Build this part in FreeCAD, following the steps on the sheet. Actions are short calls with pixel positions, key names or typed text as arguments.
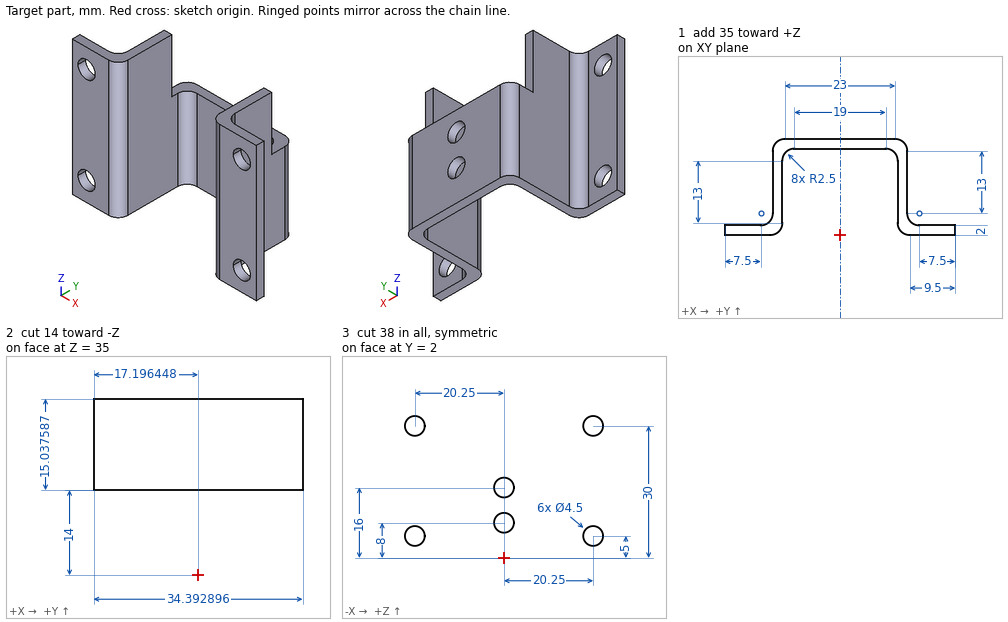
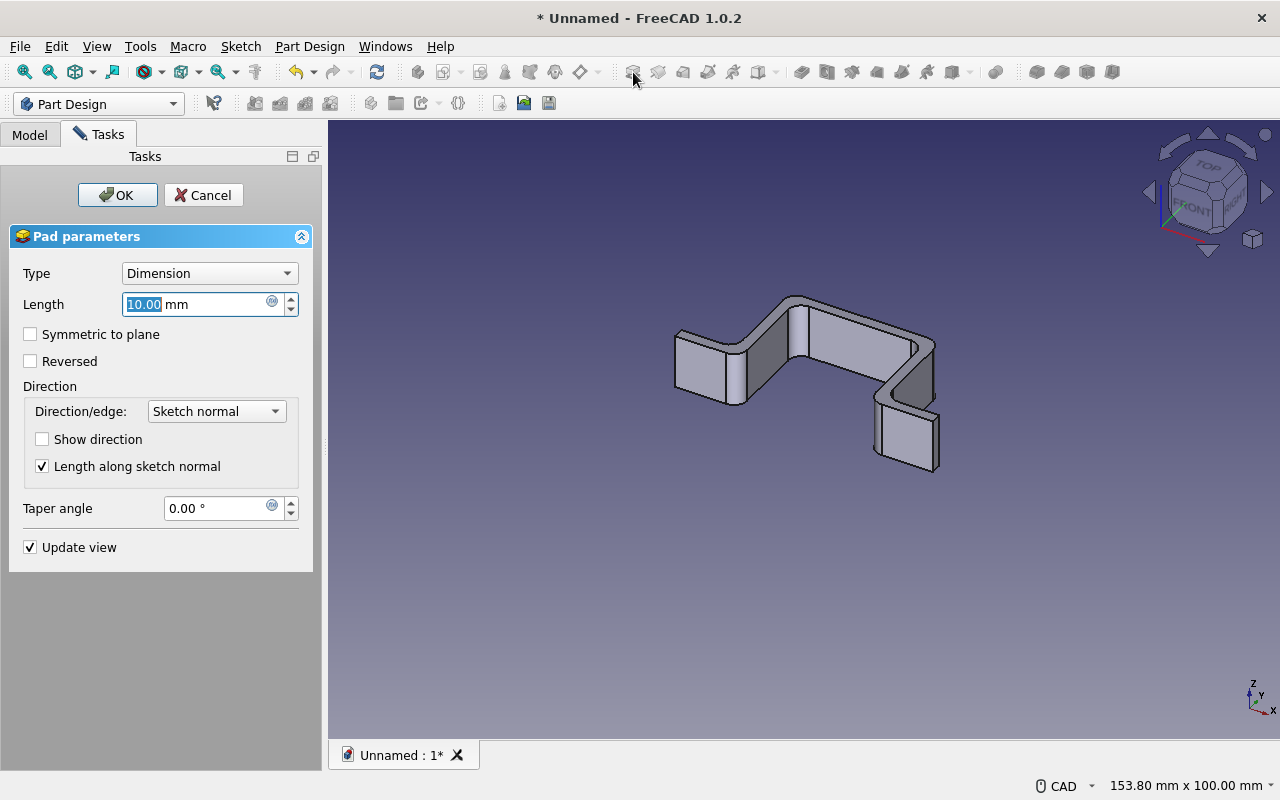
text(35)
key(Tab)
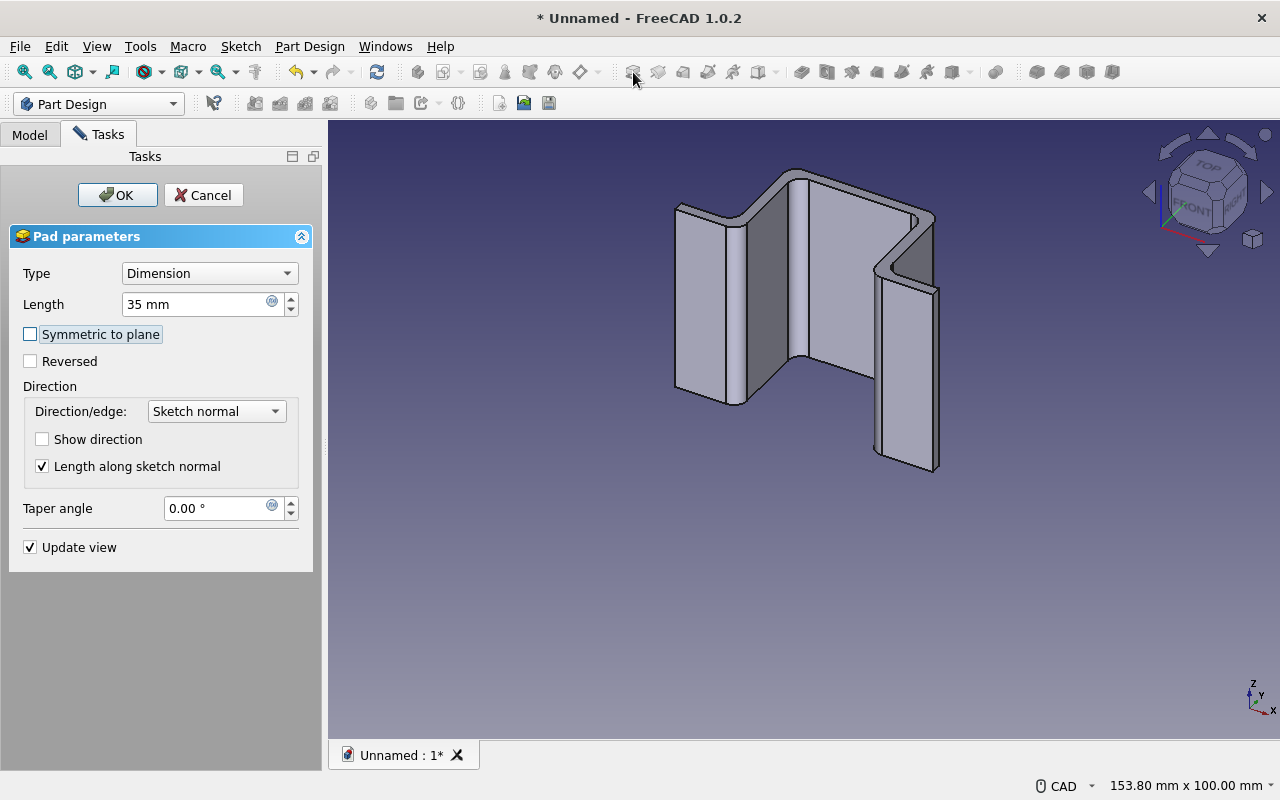
click(118, 195)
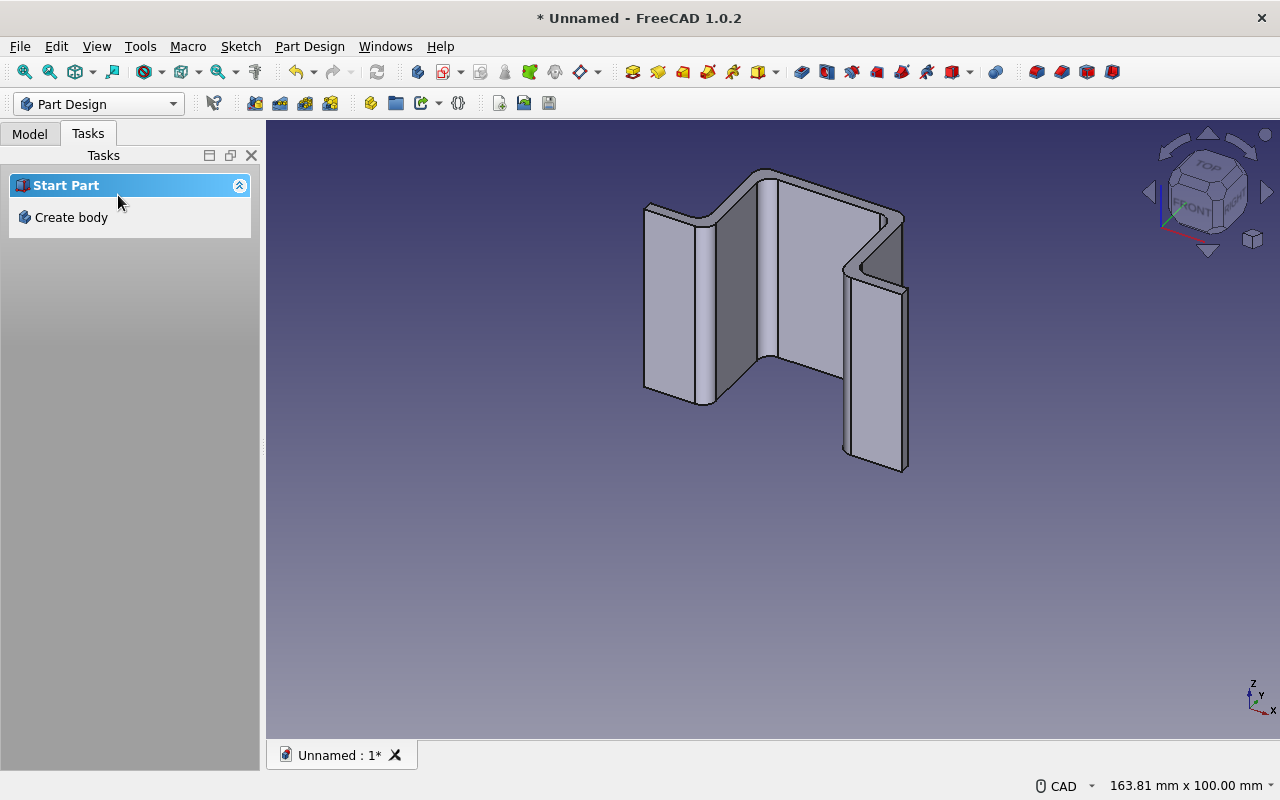
key(0)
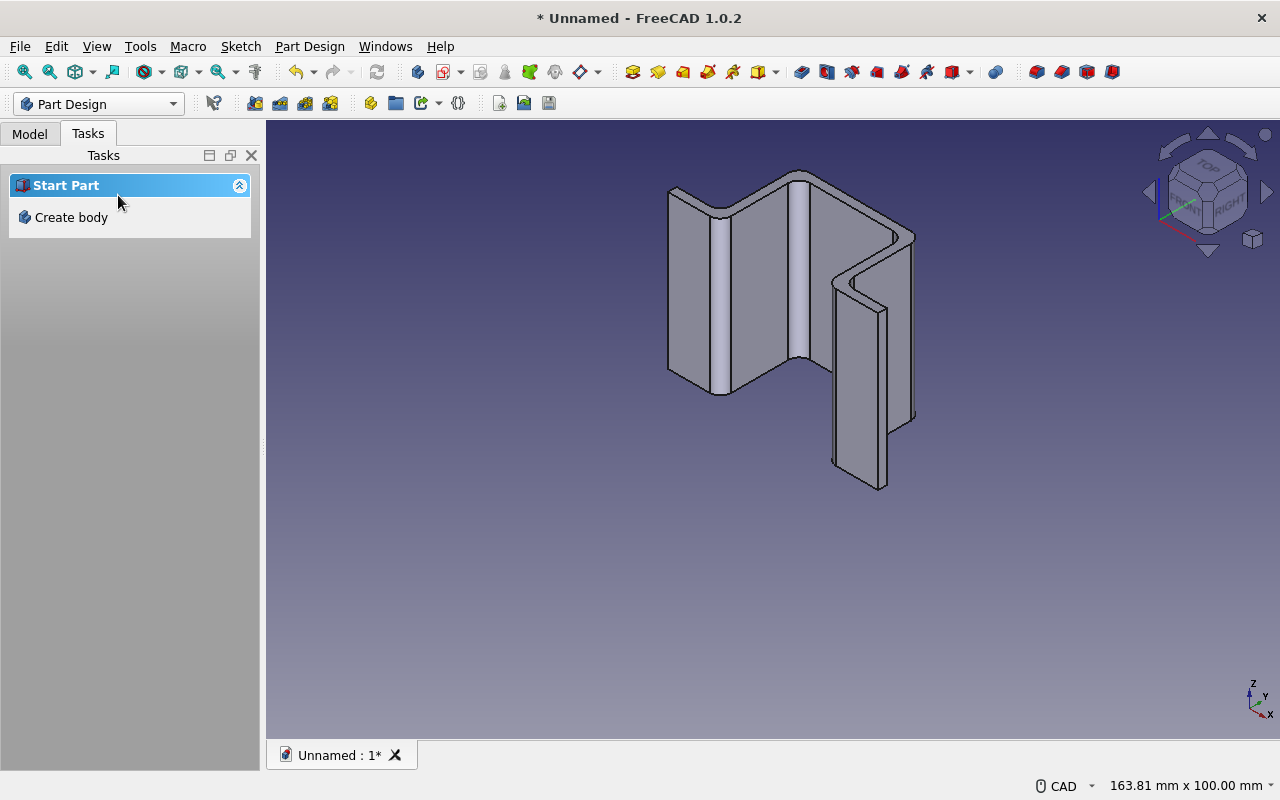
key(2)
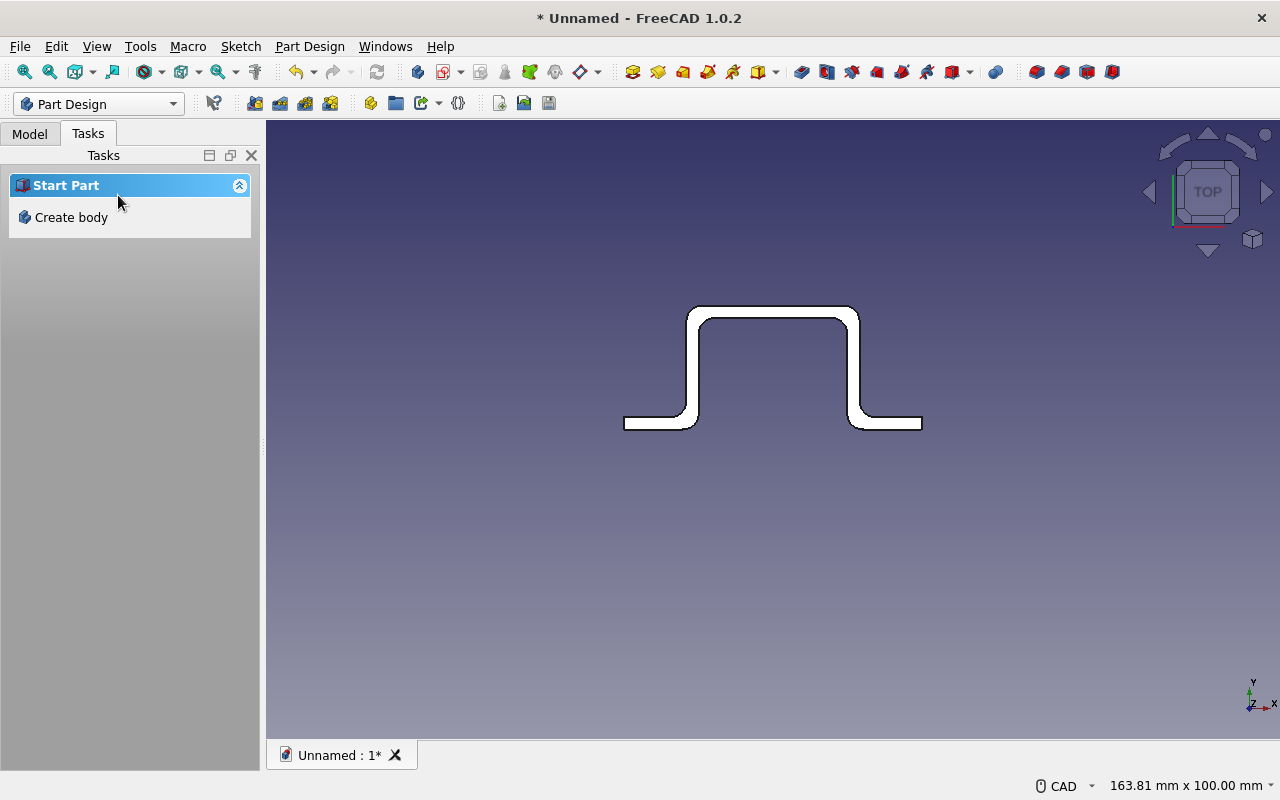
click(25, 72)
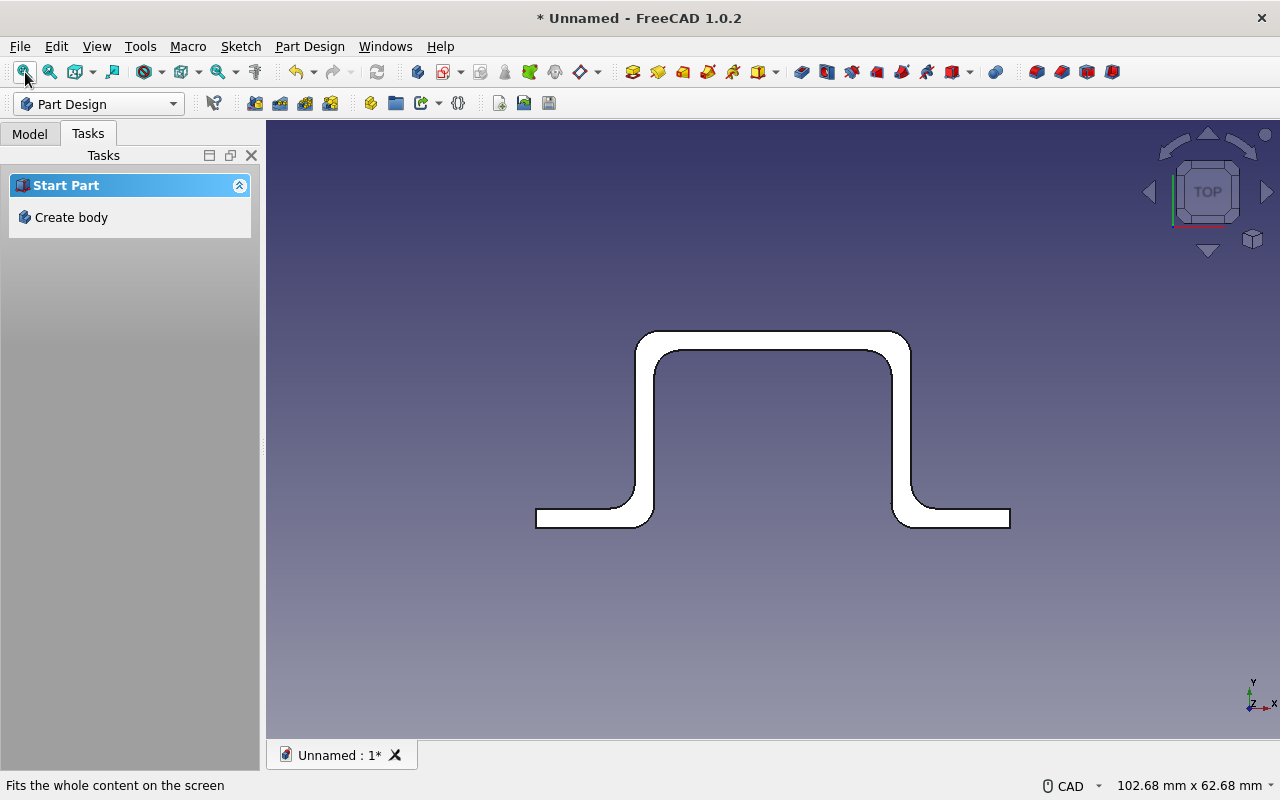
click(908, 513)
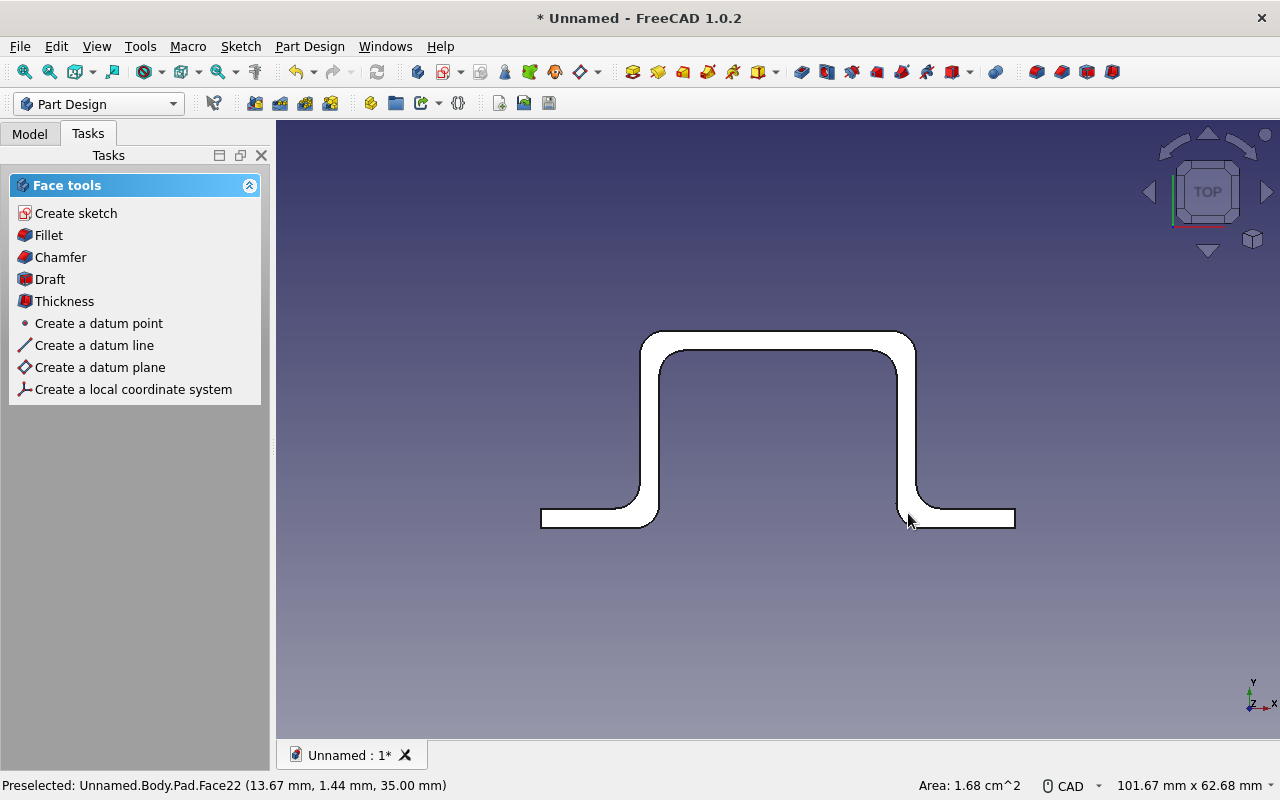
click(442, 72)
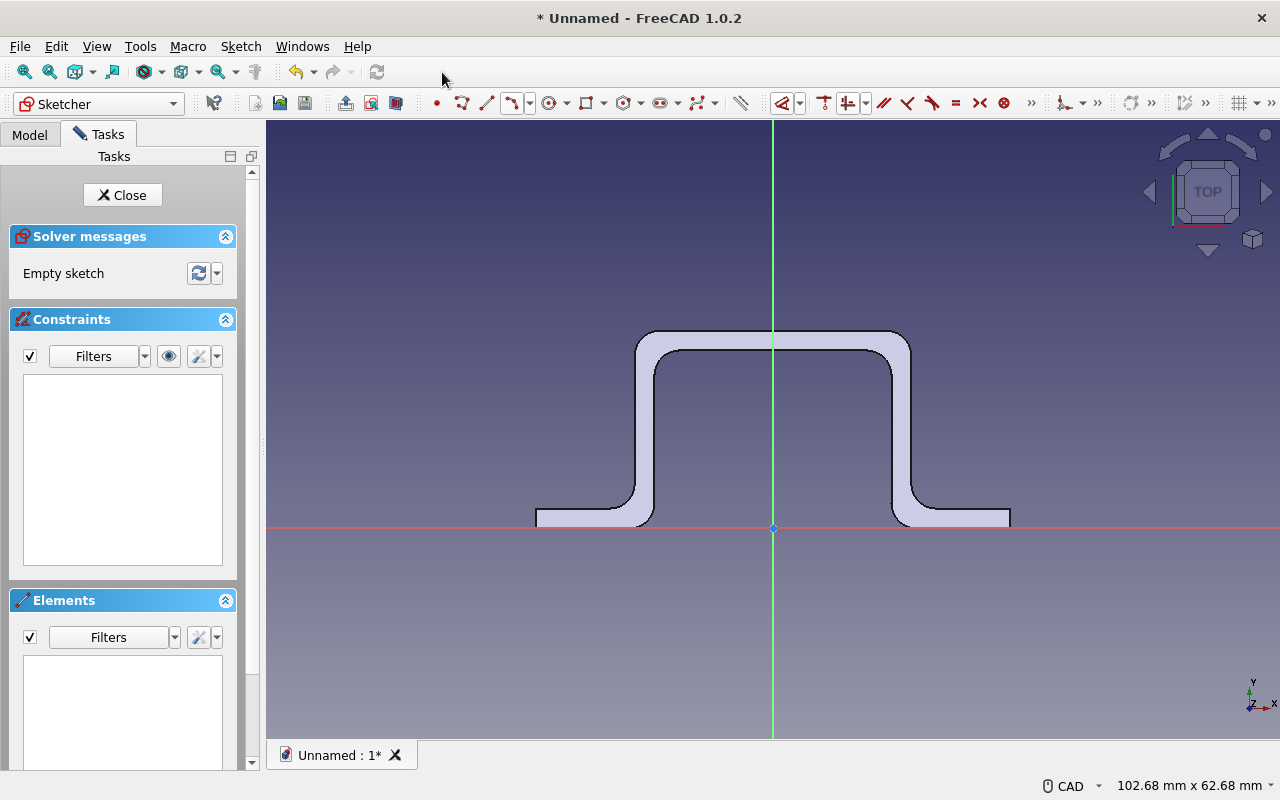
scroll(912, 294, up, 2)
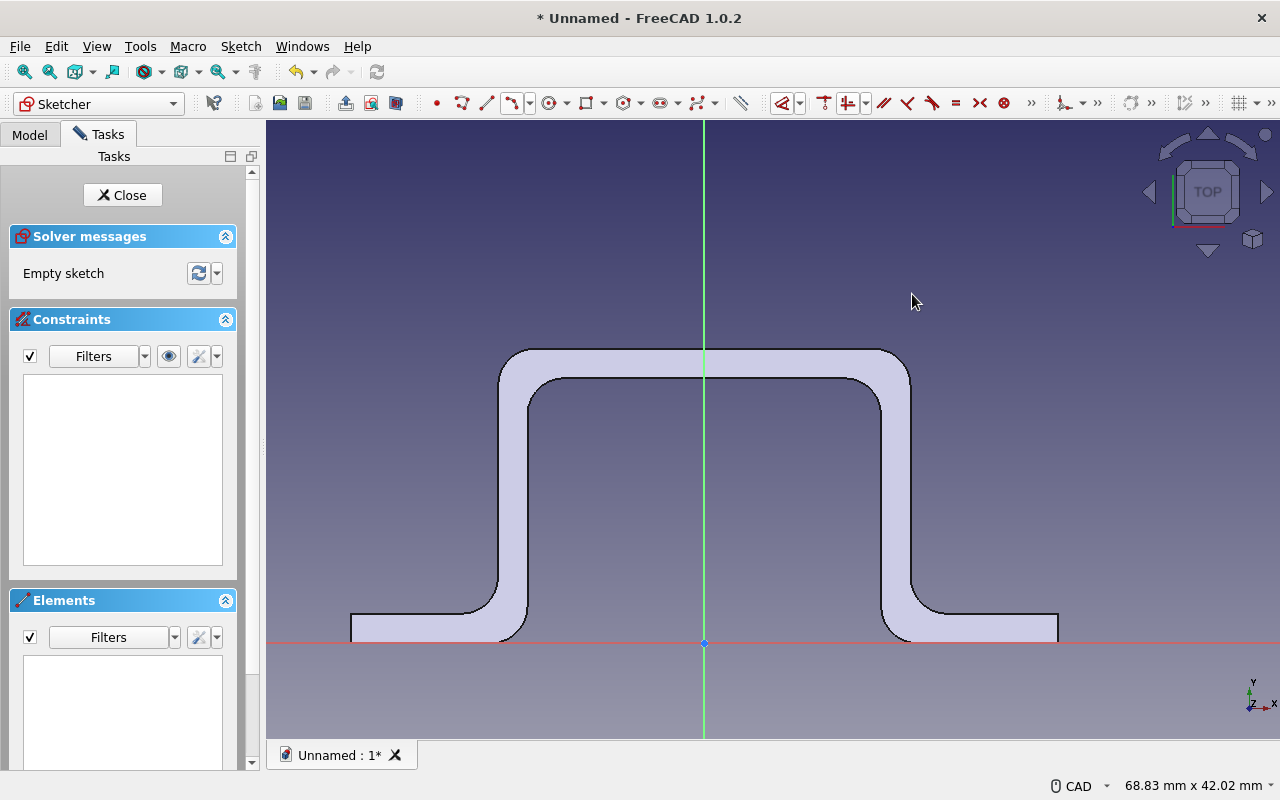
click(586, 104)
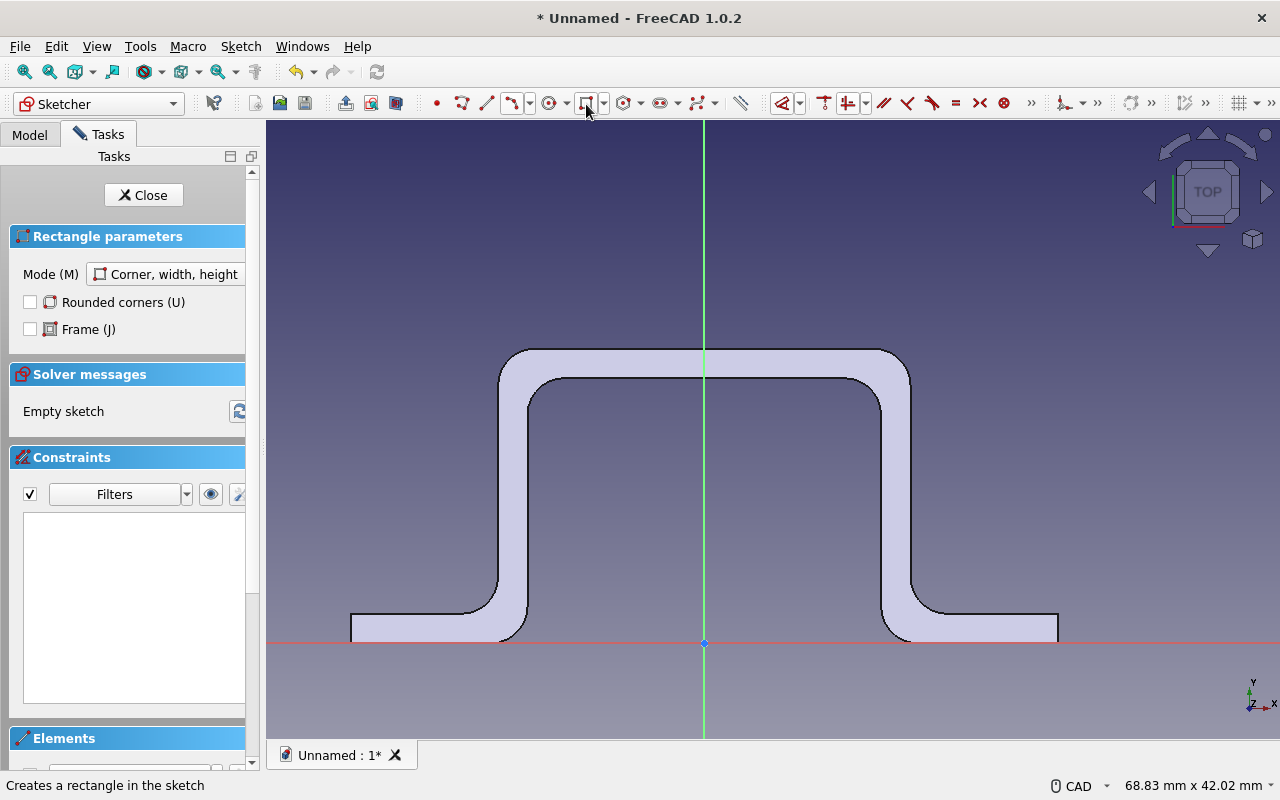
click(451, 216)
click(958, 437)
key(Escape)